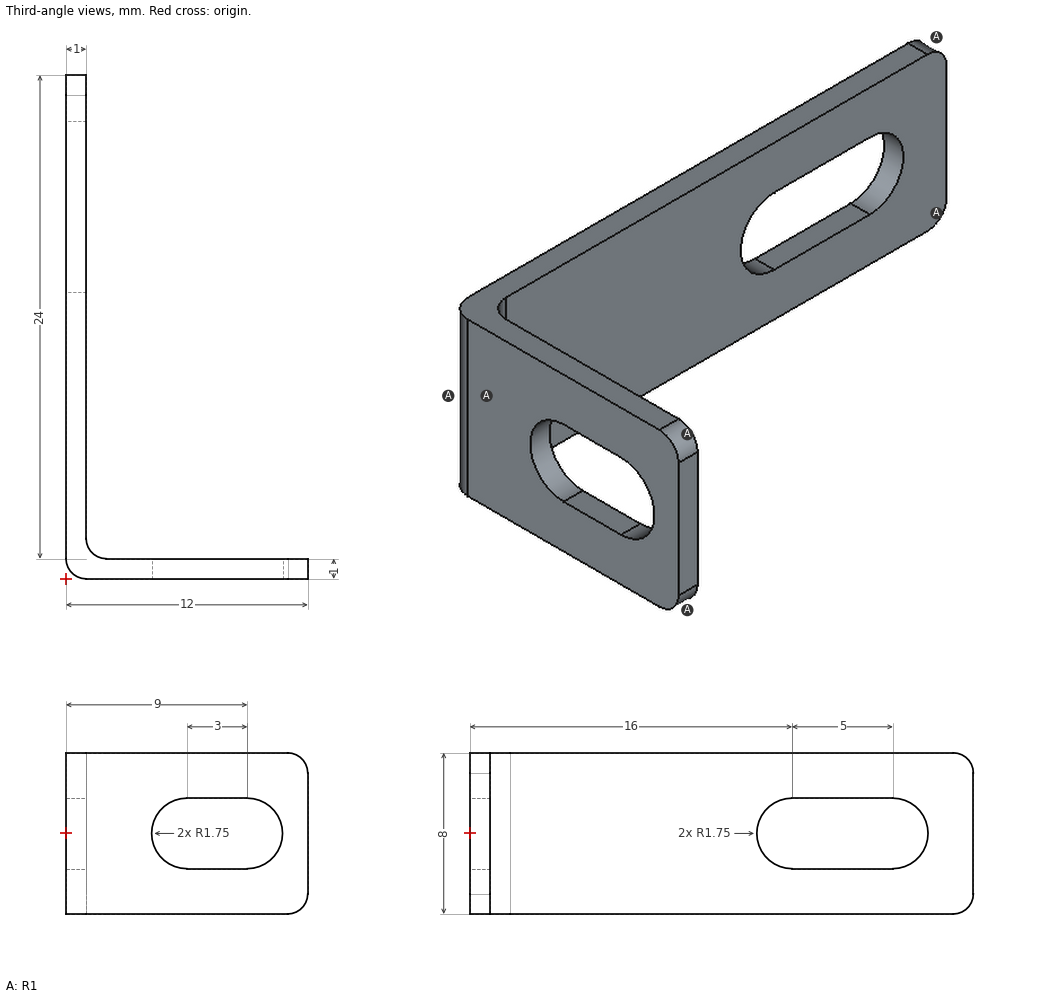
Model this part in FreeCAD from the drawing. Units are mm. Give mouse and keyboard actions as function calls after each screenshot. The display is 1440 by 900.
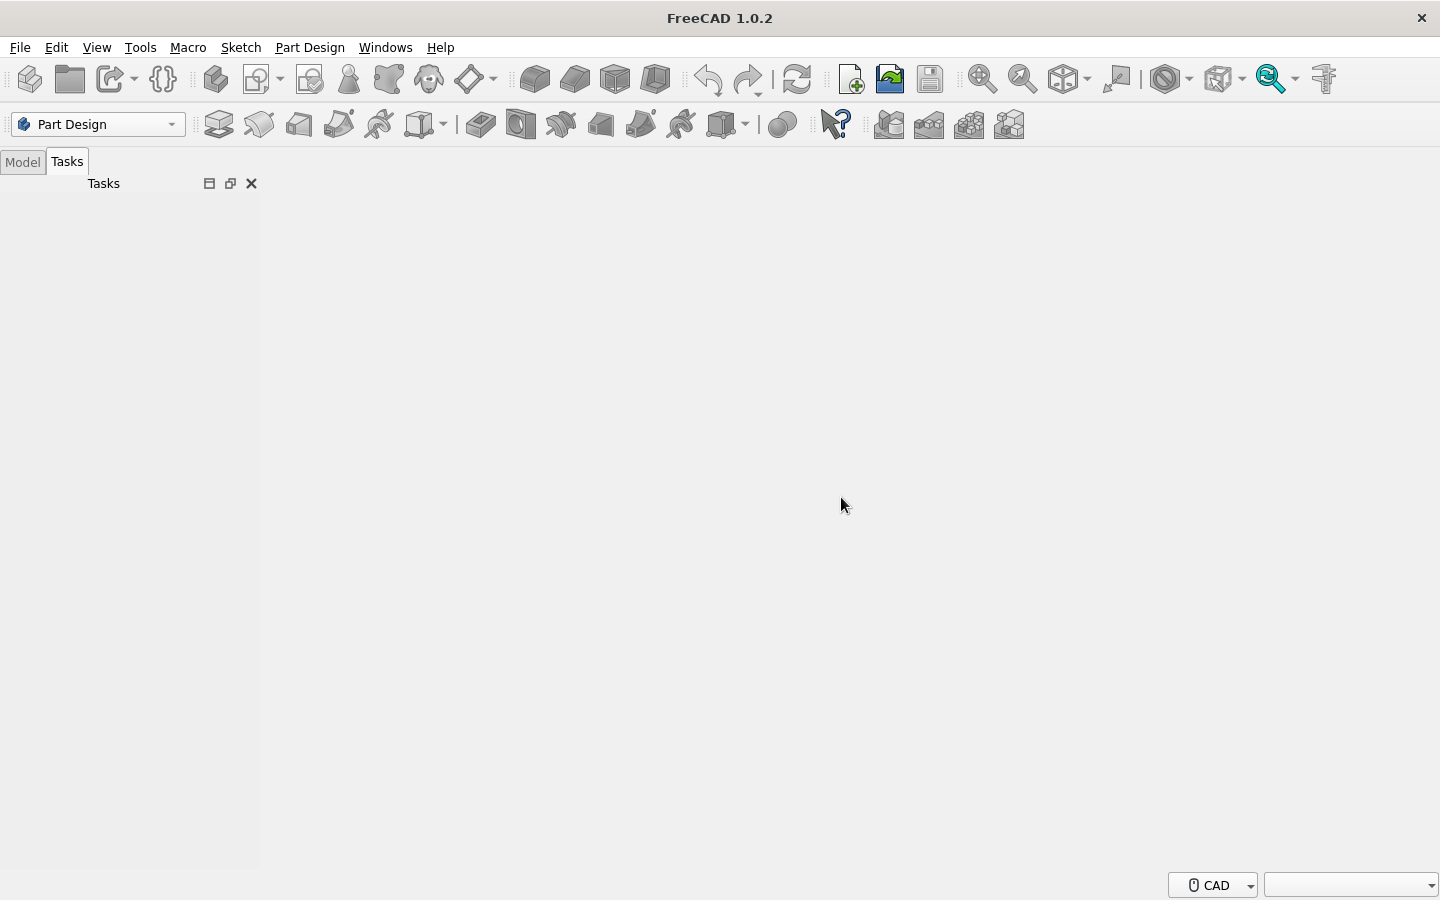
key(ctrl+n)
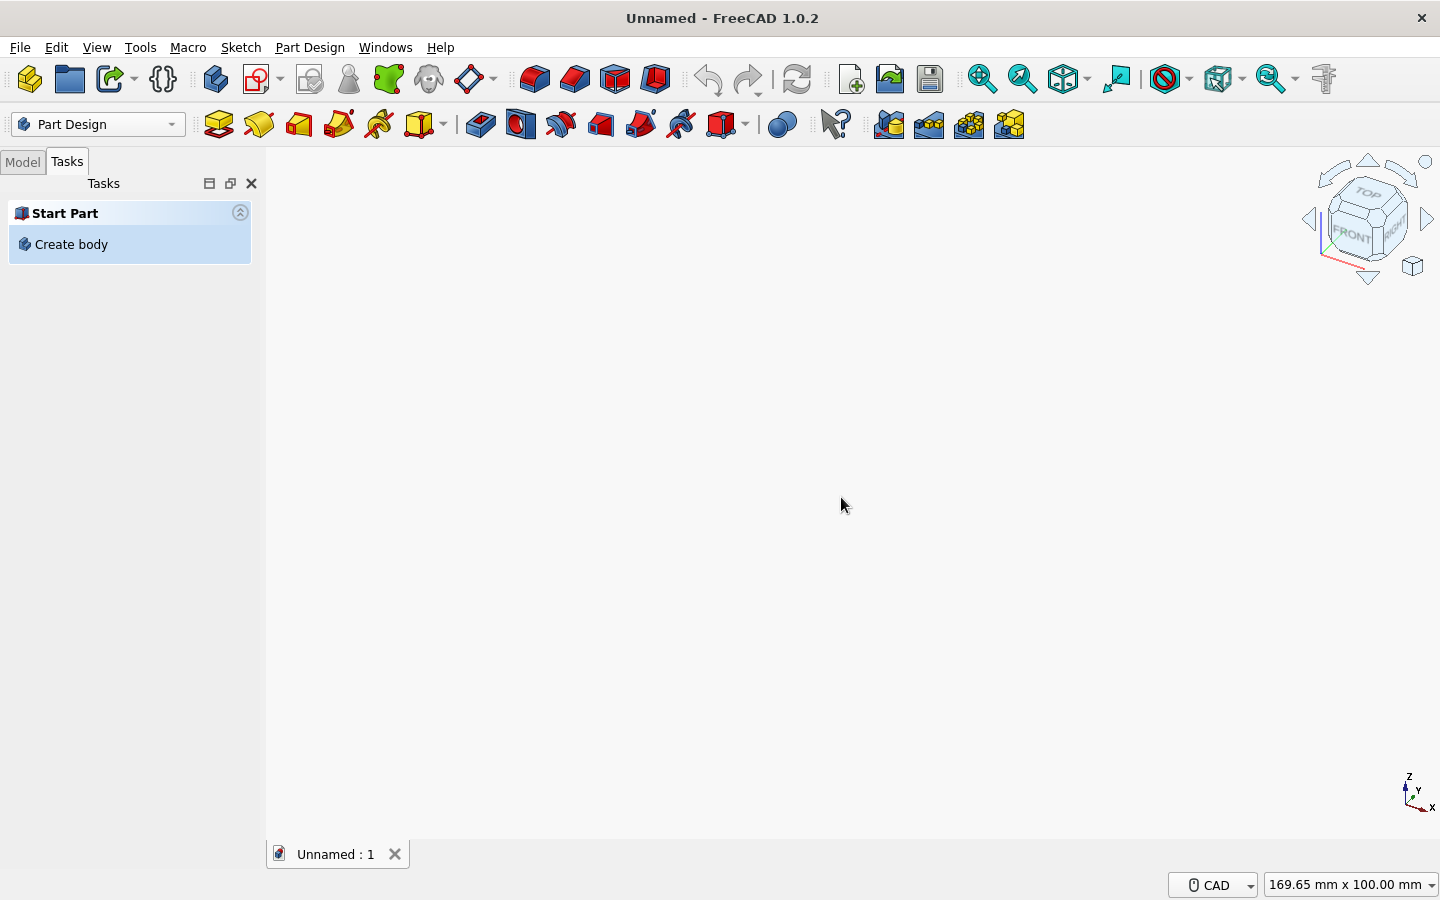
click(256, 80)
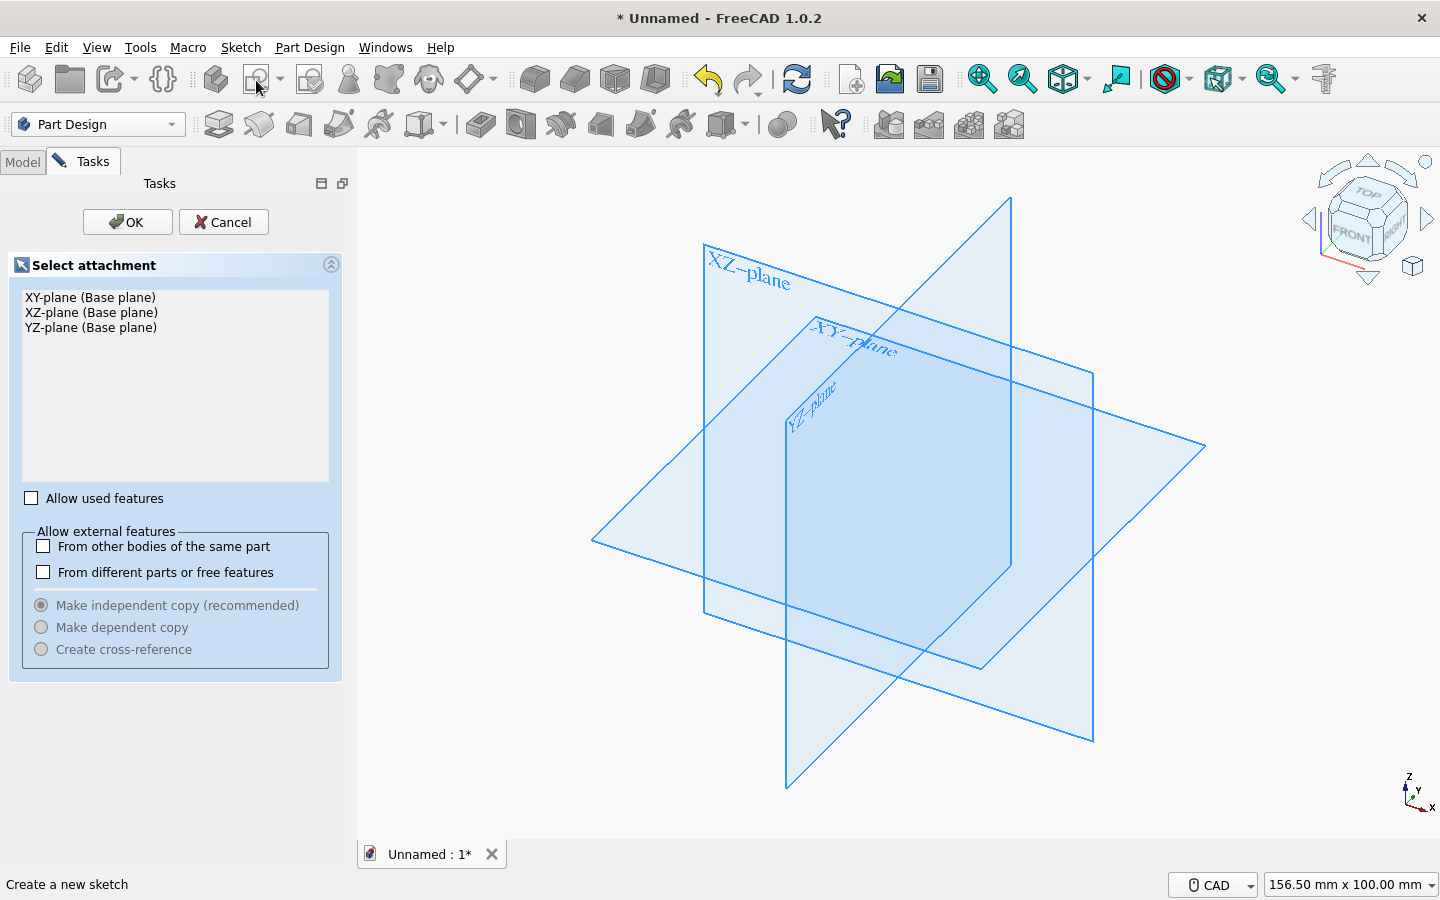
click(82, 298)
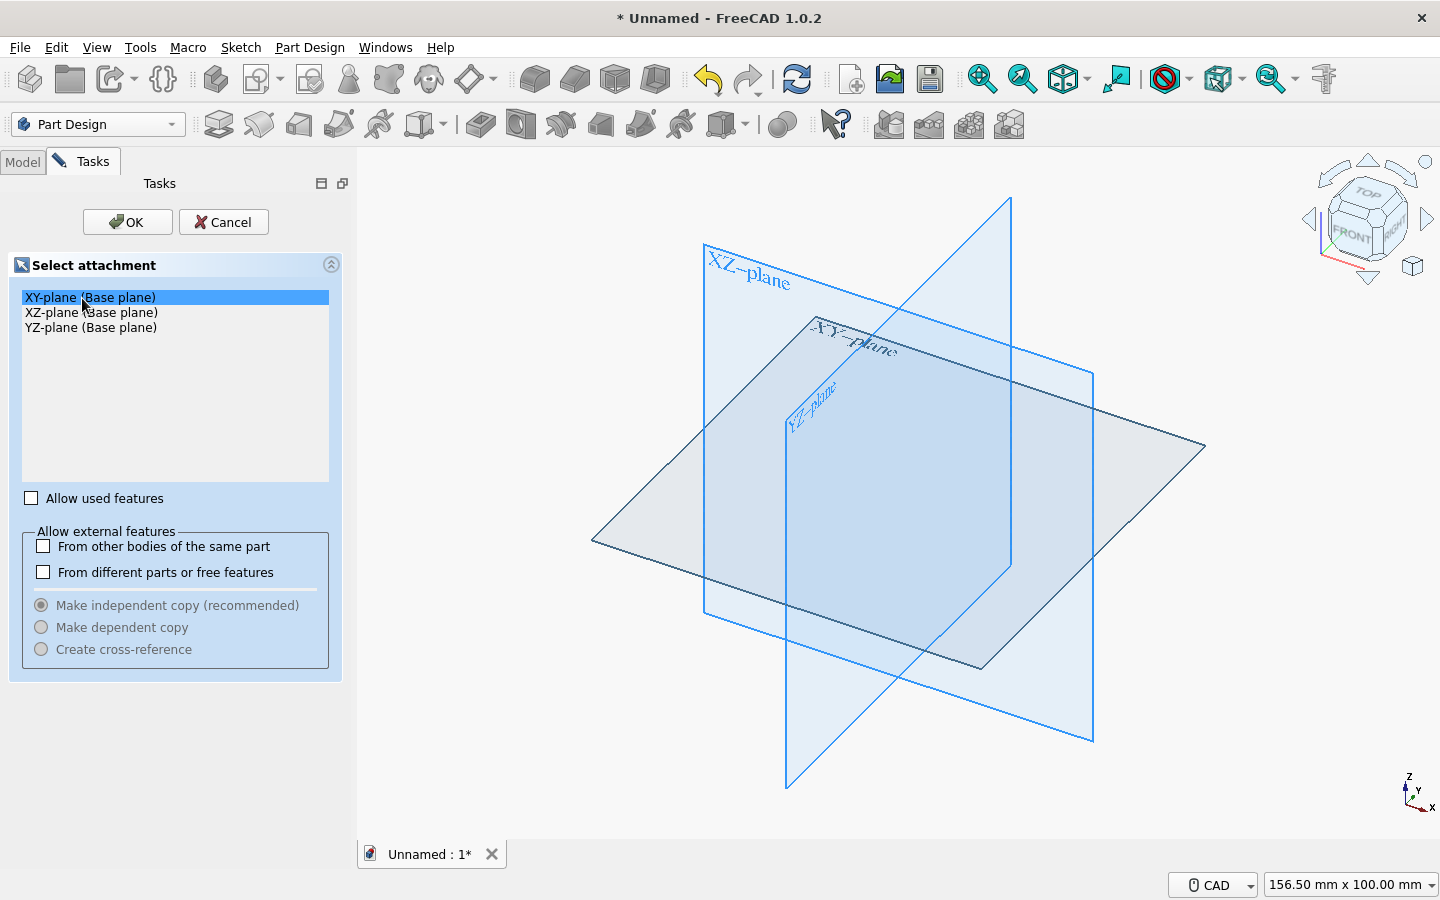
click(128, 222)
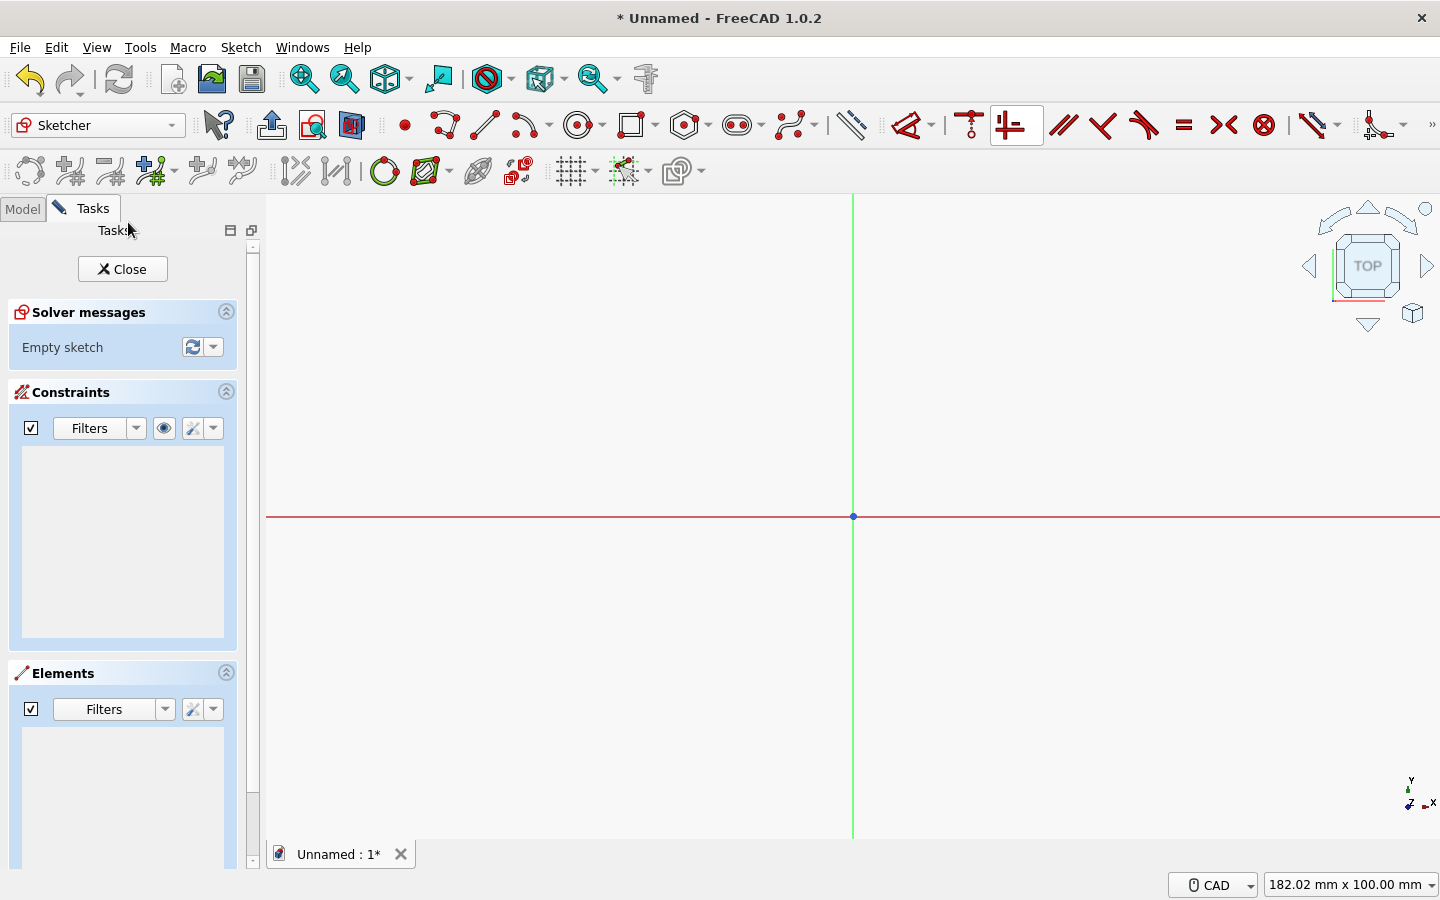
scroll(954, 389, up, 5)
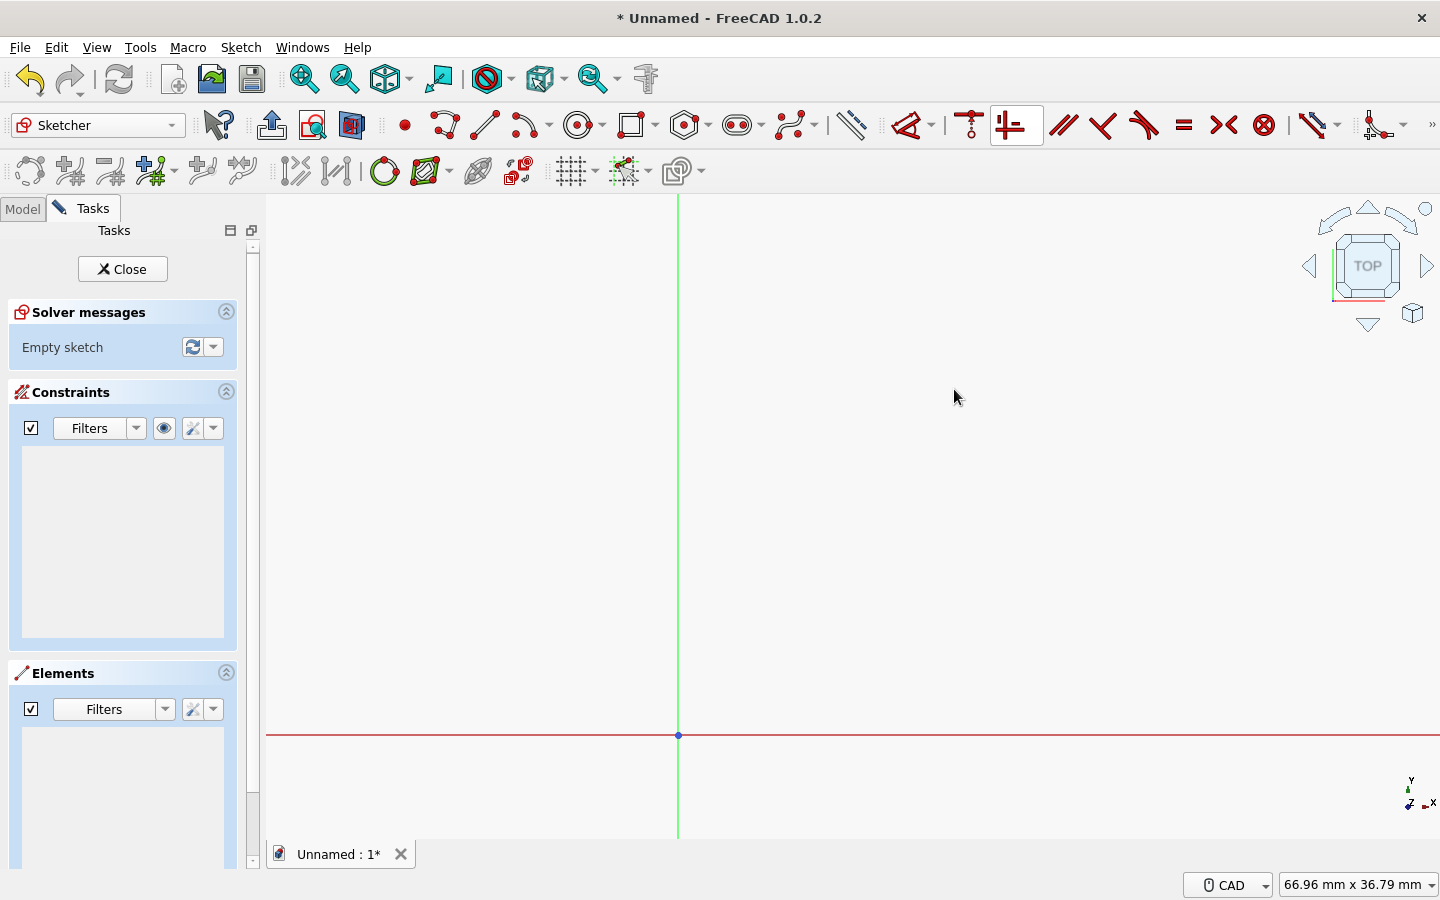
click(446, 126)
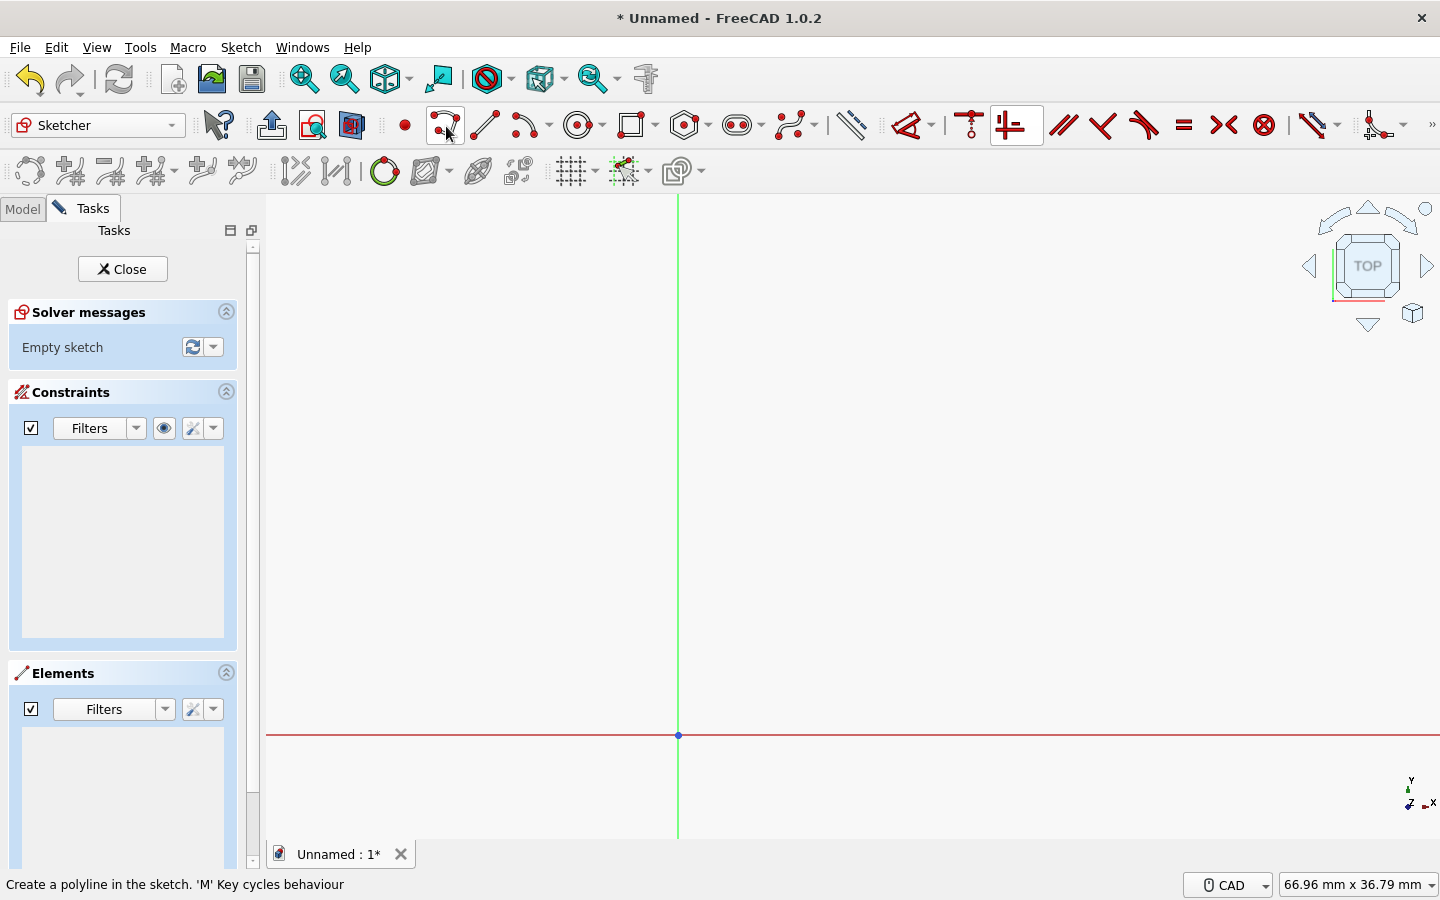
click(678, 735)
click(889, 726)
click(889, 718)
click(696, 718)
click(696, 297)
click(687, 297)
click(678, 735)
key(Escape)
key(Escape)